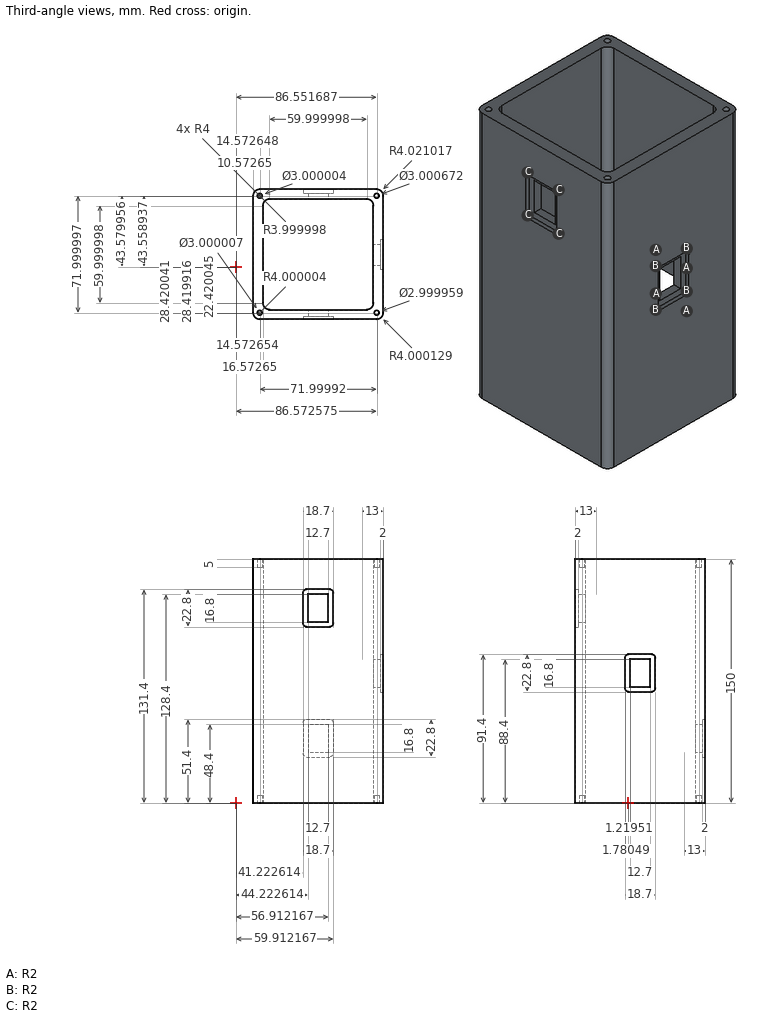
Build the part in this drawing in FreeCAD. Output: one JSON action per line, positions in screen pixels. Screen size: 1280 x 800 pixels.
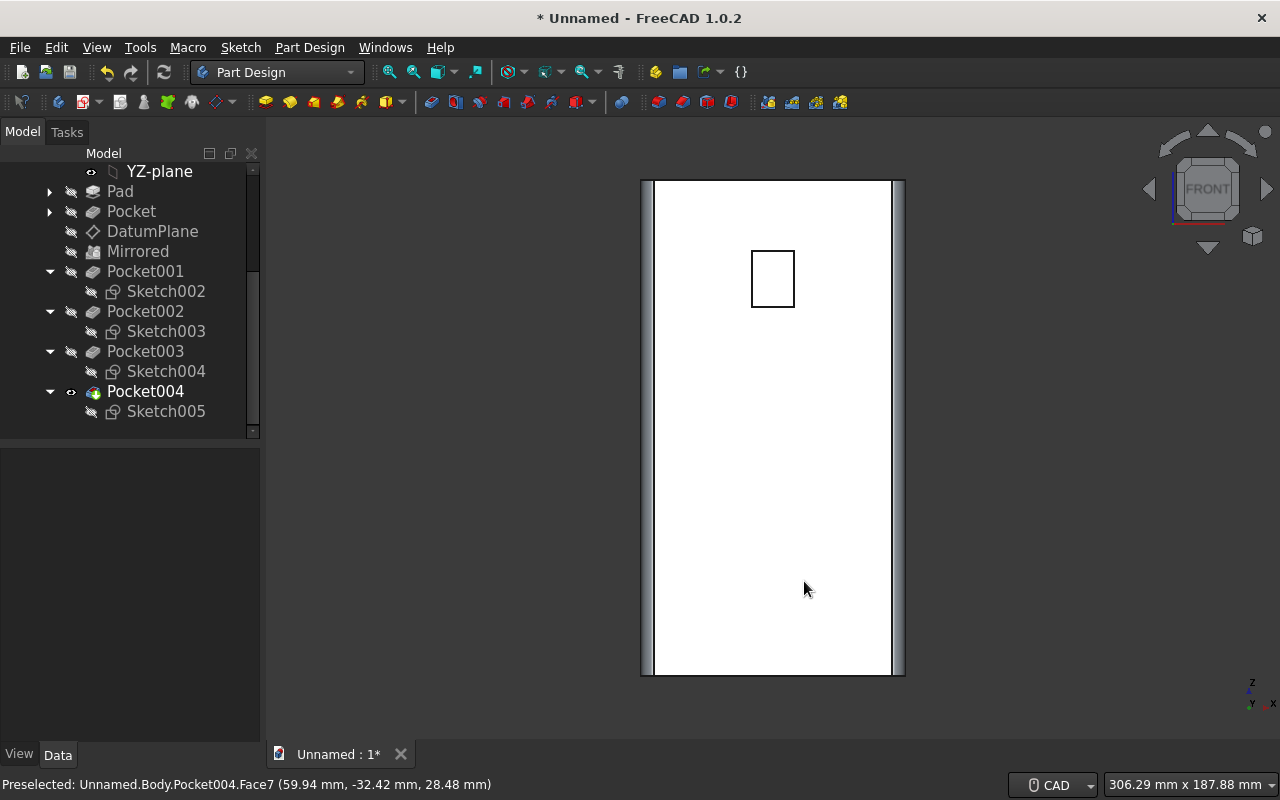
{"action": "key", "text": "3"}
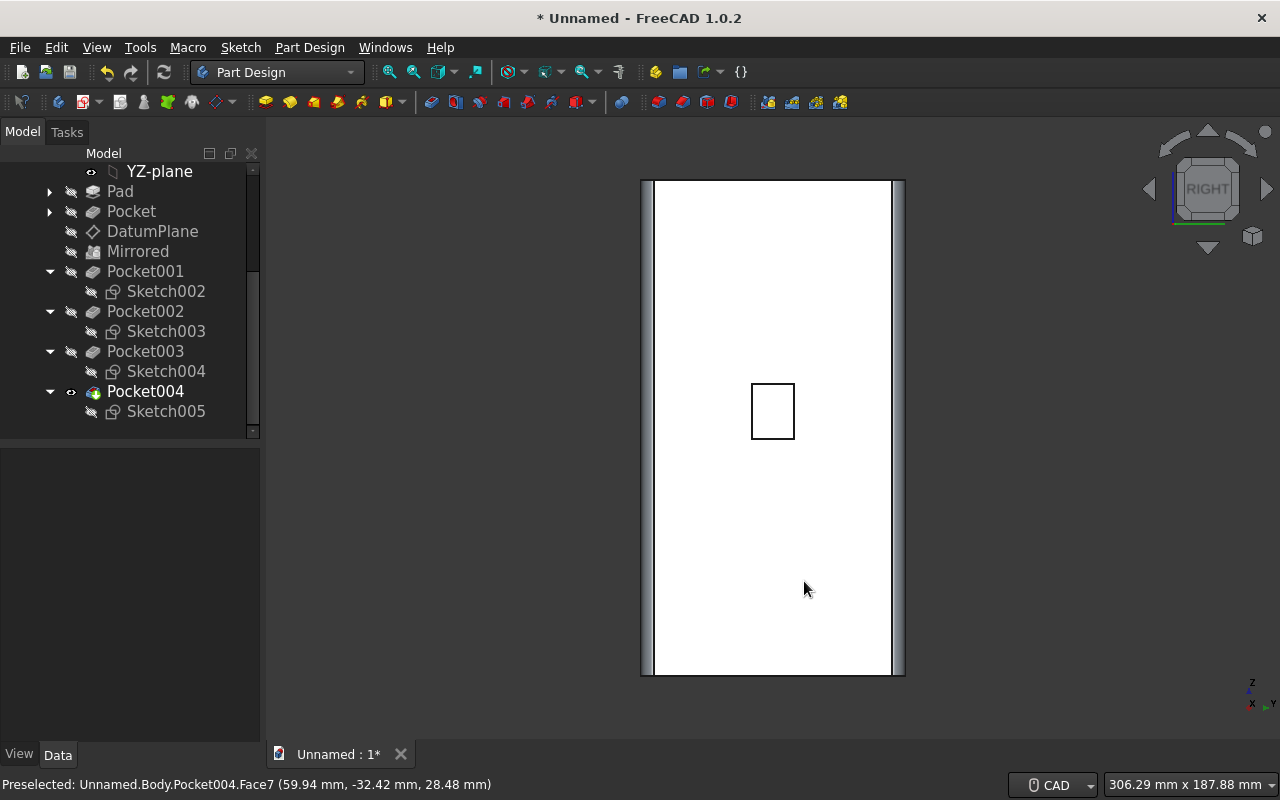
{"action": "scroll", "coordinate": [902, 581], "scroll_direction": "up", "scroll_amount": 9}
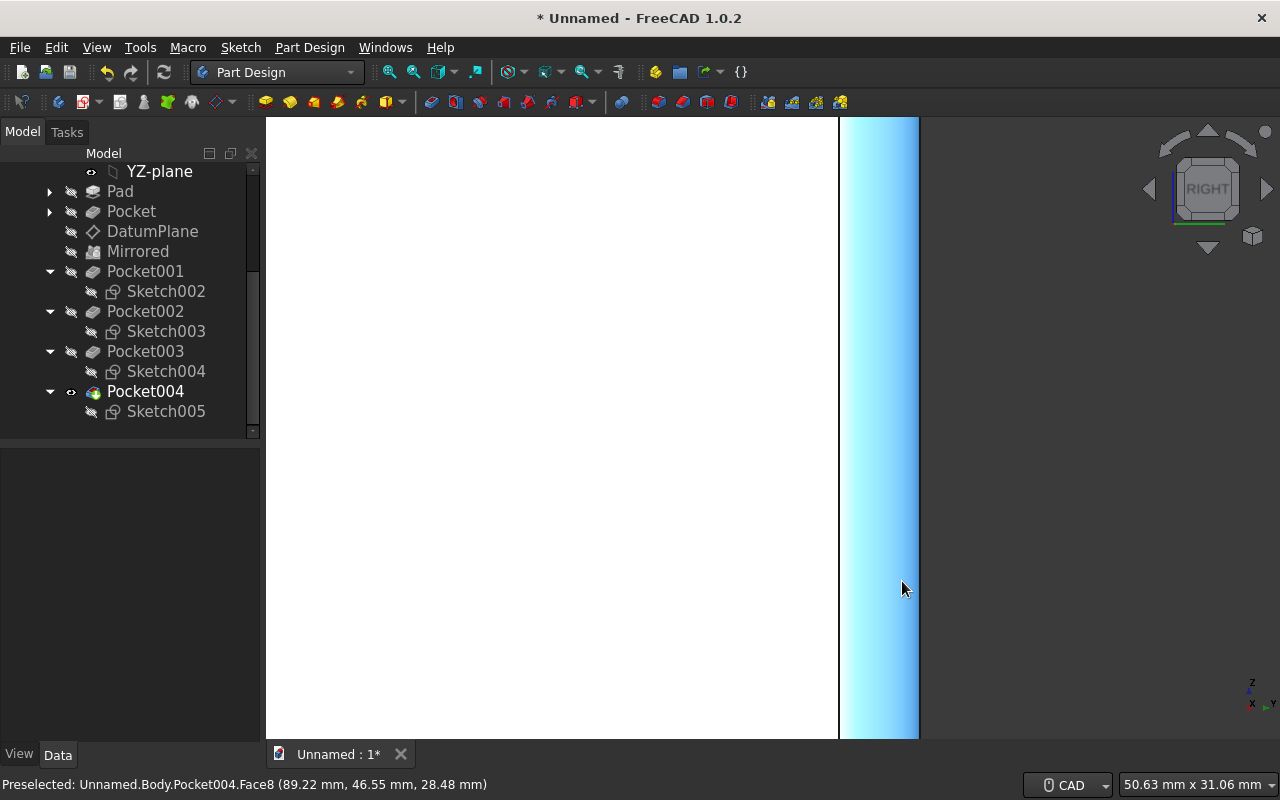
{"action": "key", "text": "v f"}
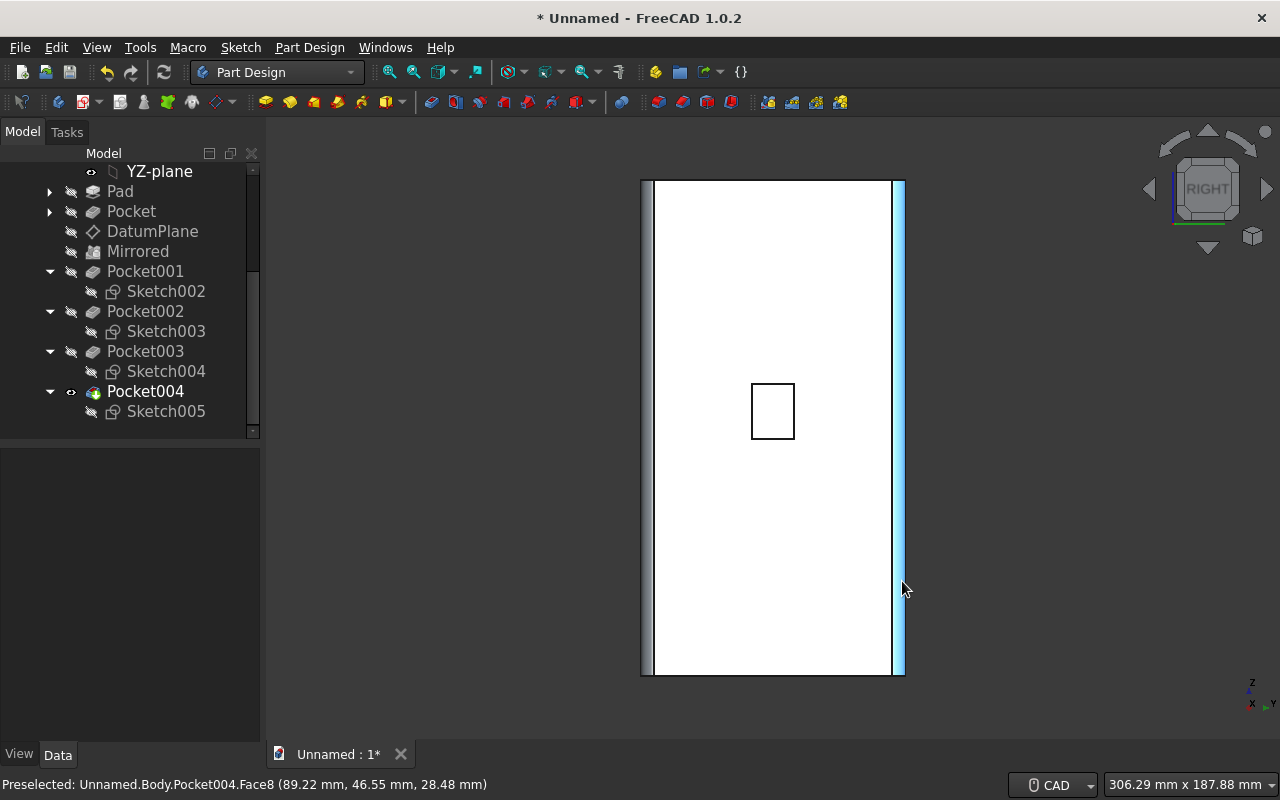
{"action": "key", "text": "5"}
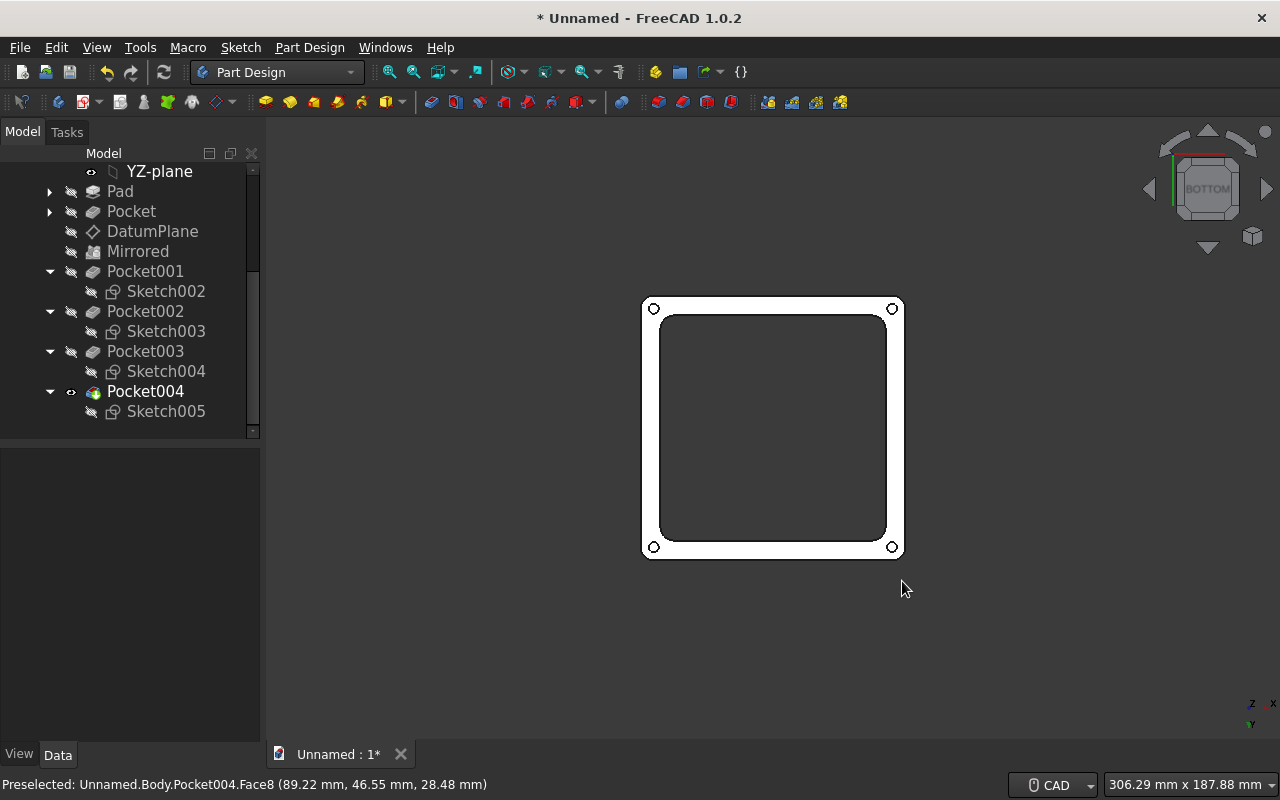
{"action": "left_click", "coordinate": [390, 72]}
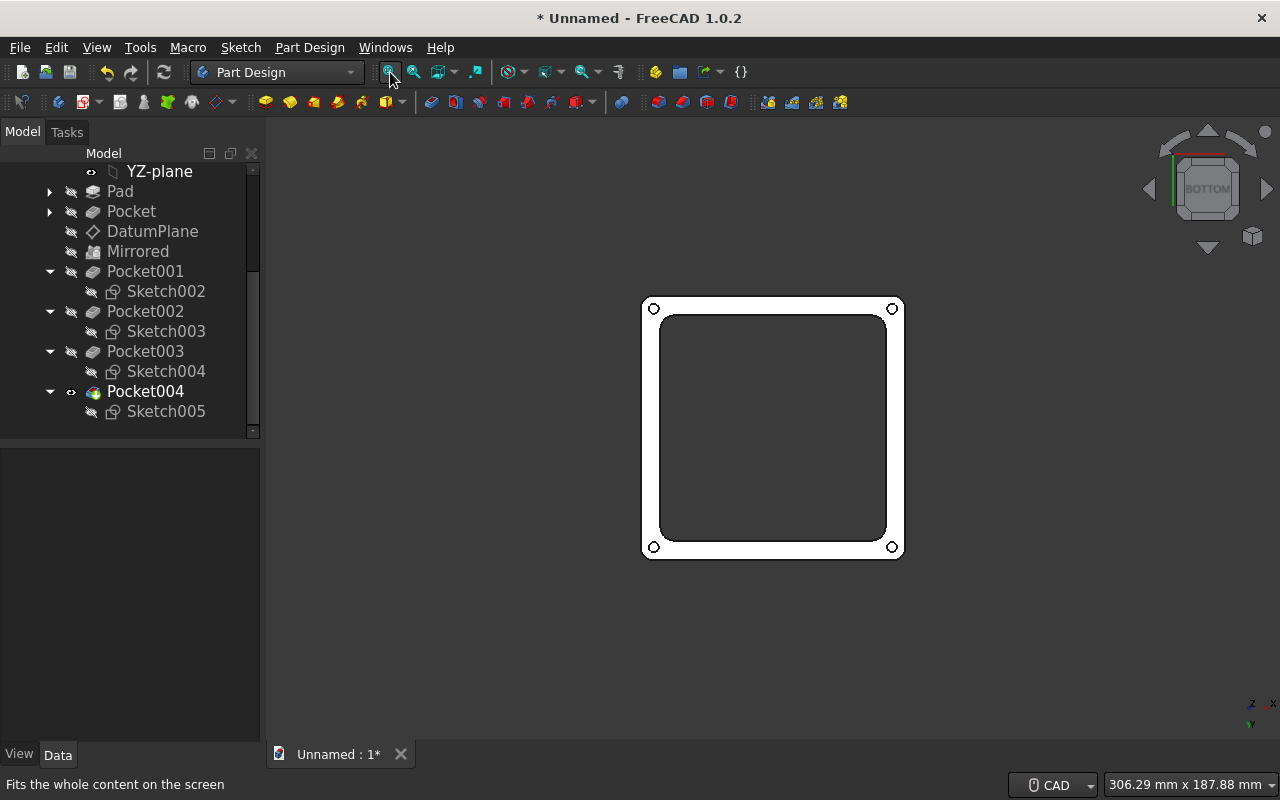
{"action": "scroll", "coordinate": [804, 556], "scroll_direction": "up", "scroll_amount": 9}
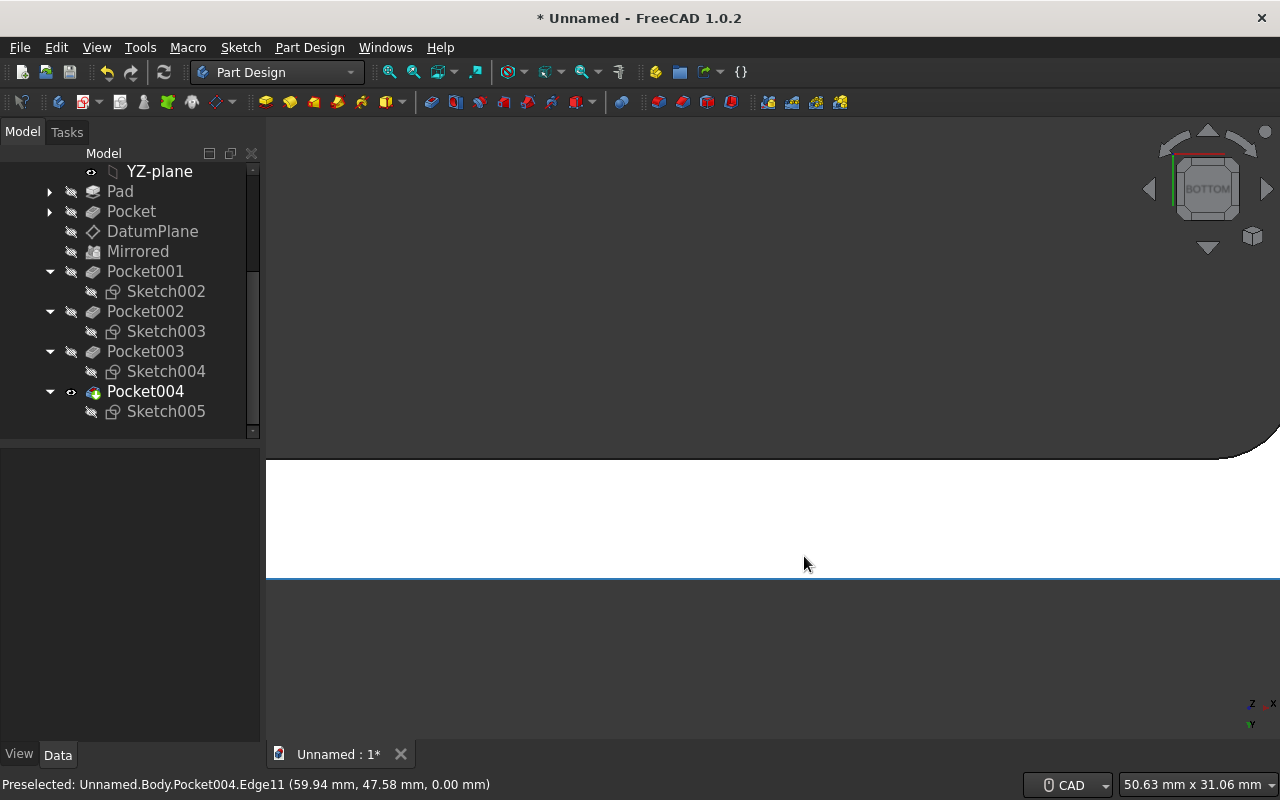
{"action": "left_click", "coordinate": [390, 72]}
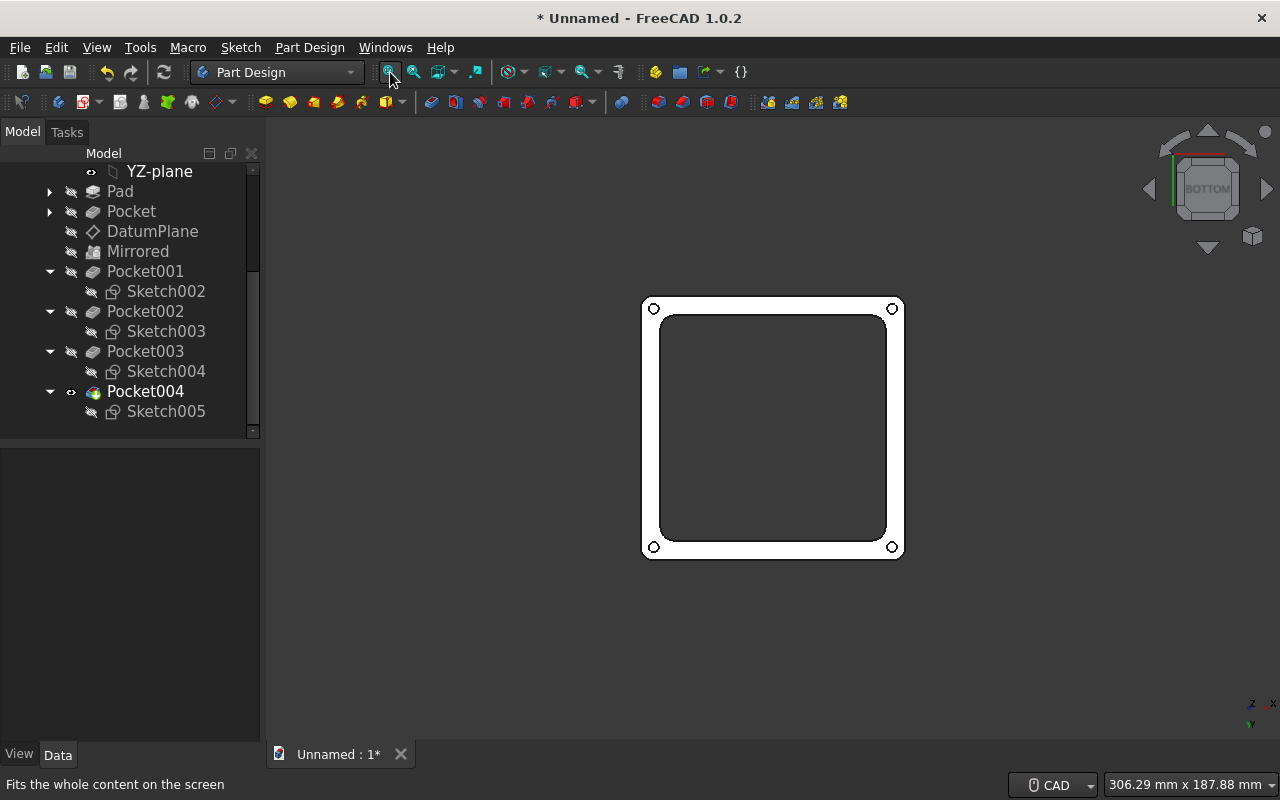
{"action": "key", "text": "4"}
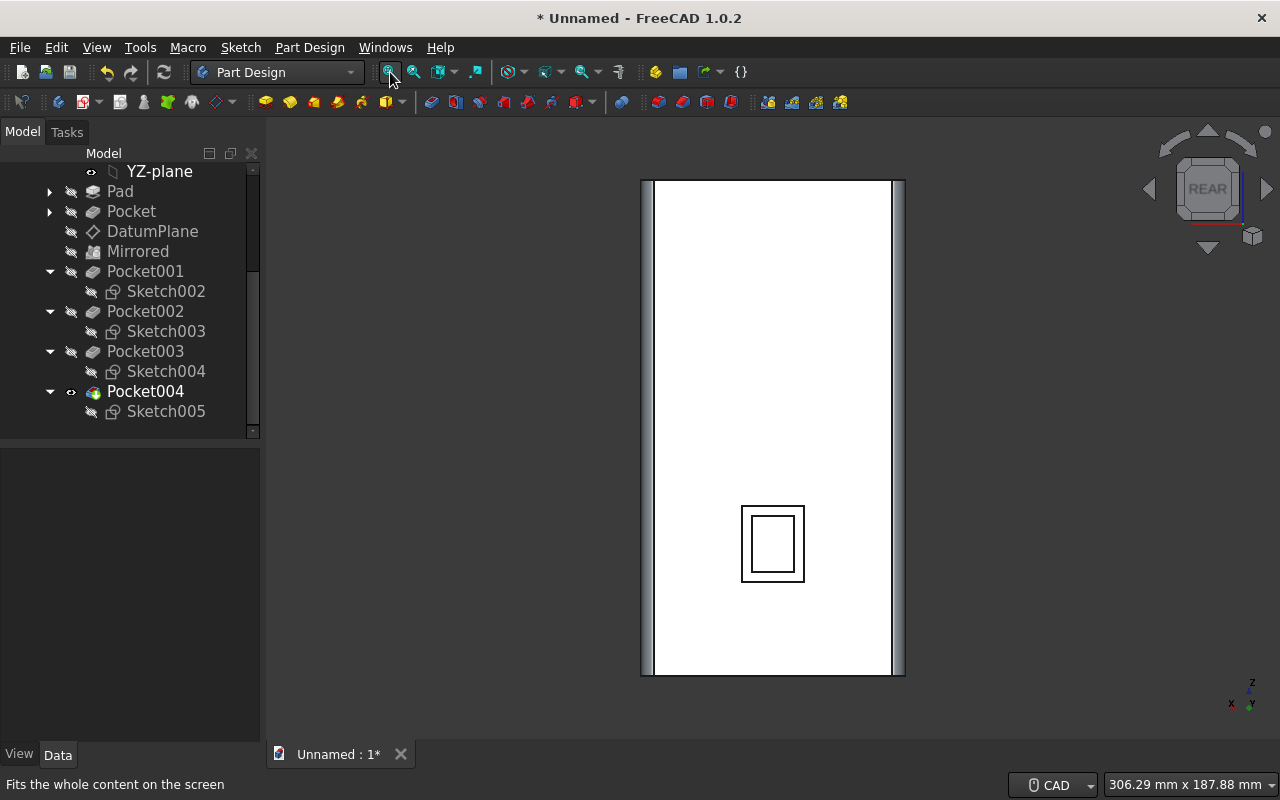
{"action": "scroll", "coordinate": [742, 581], "scroll_direction": "up", "scroll_amount": 9}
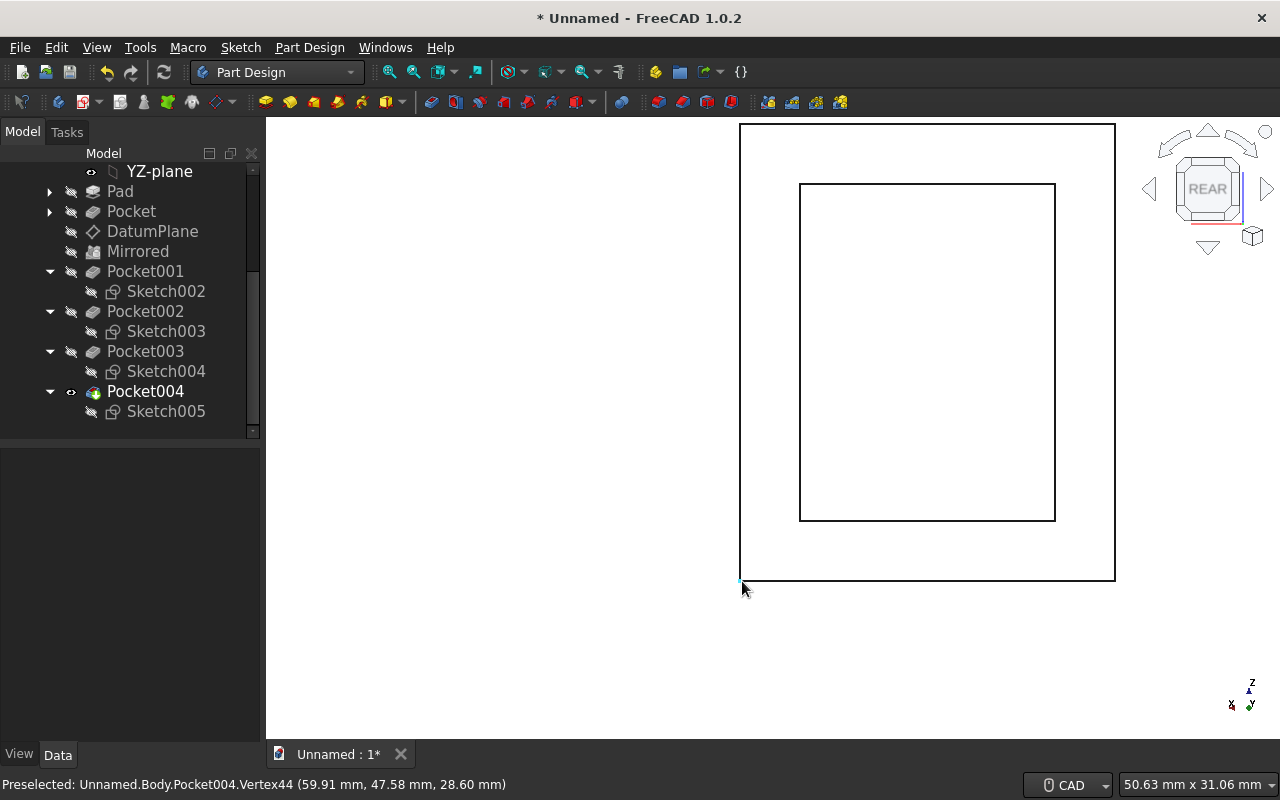
{"action": "key", "text": "v f"}